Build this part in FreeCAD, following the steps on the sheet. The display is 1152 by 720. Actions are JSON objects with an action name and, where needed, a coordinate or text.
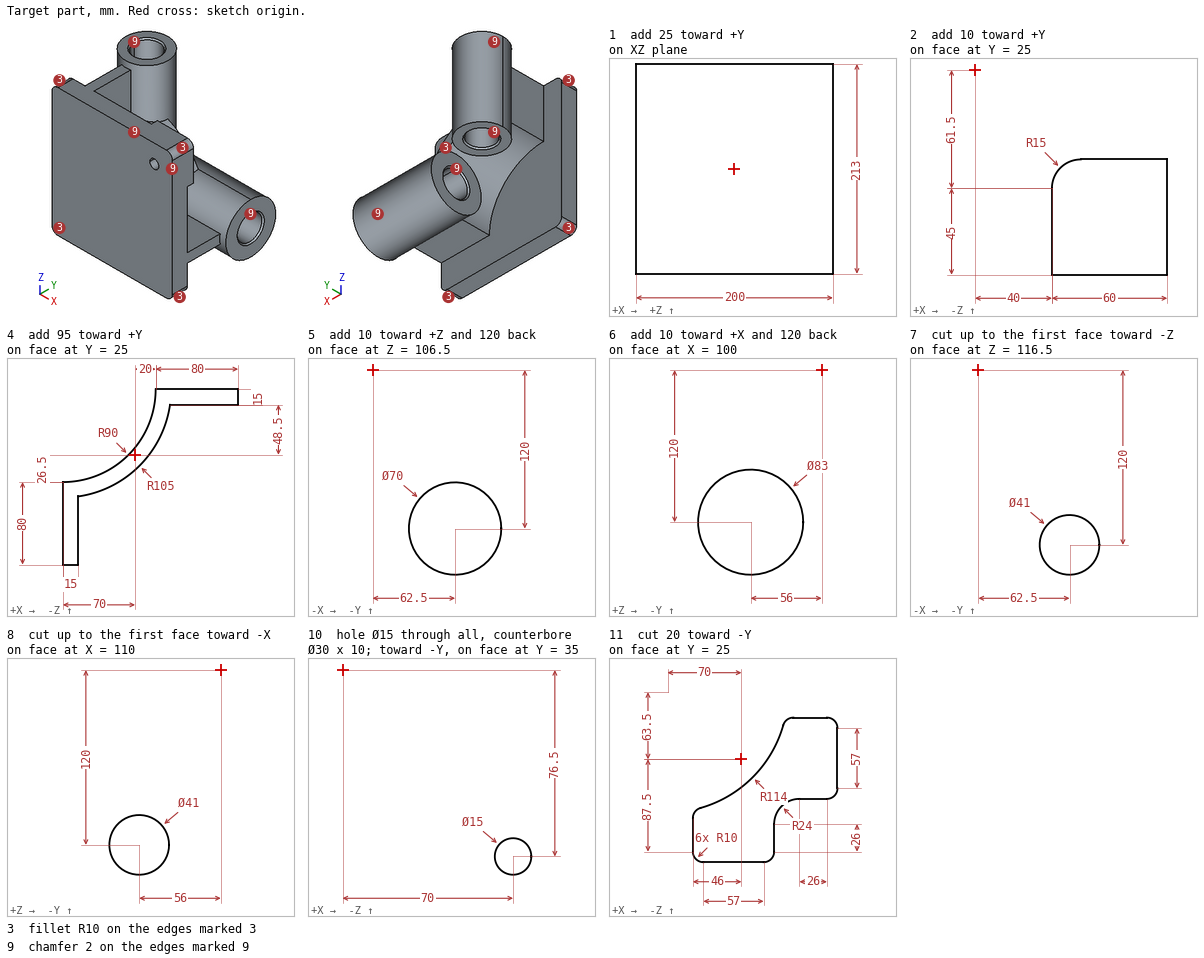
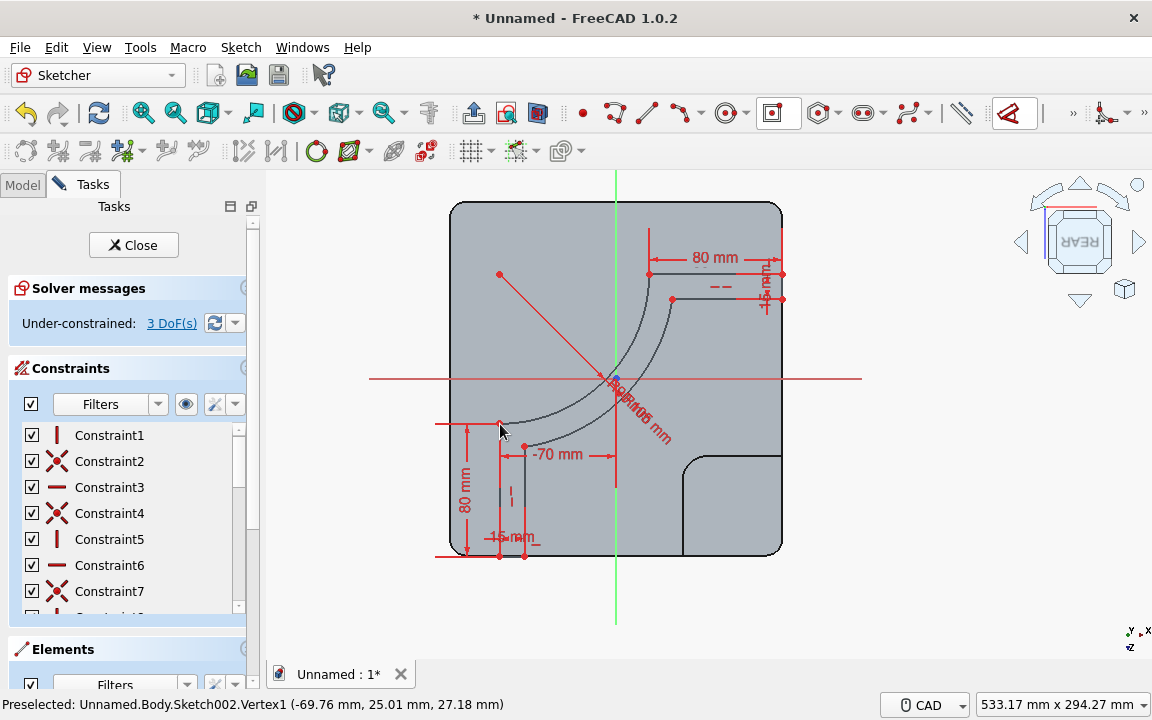
{"action": "left_click", "coordinate": [649, 274]}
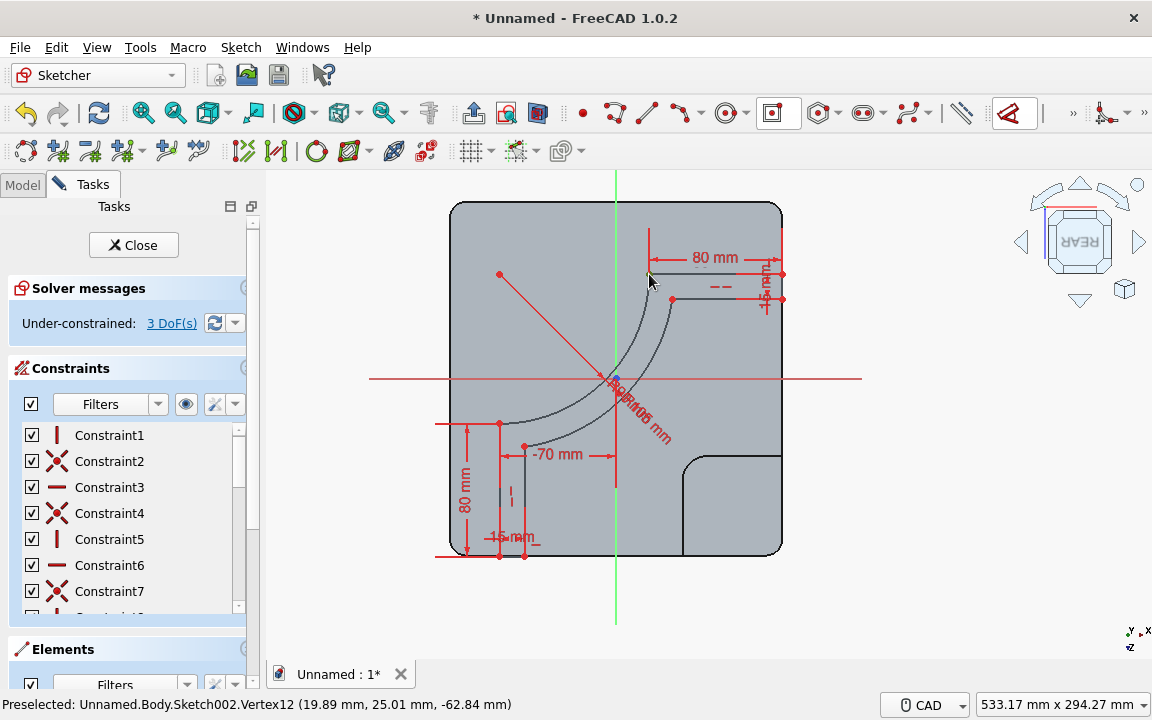
{"action": "left_click", "coordinate": [1032, 114]}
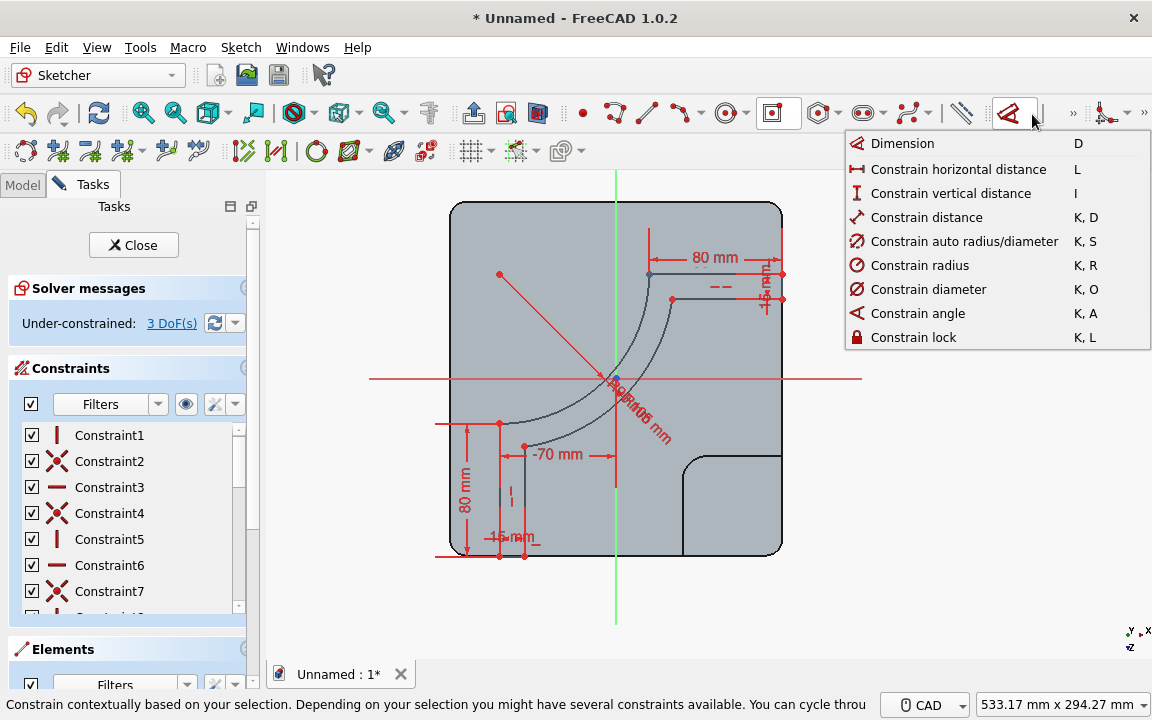
{"action": "left_click", "coordinate": [998, 169]}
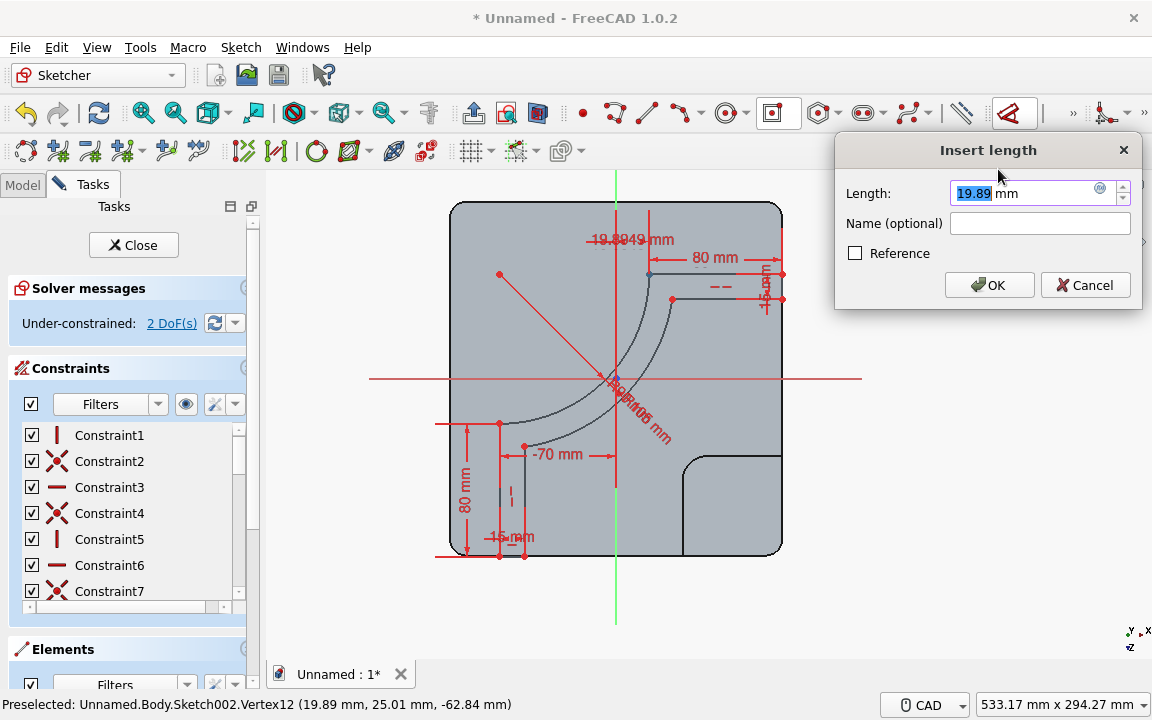
{"action": "type", "text": "20"}
{"action": "key", "text": "Return"}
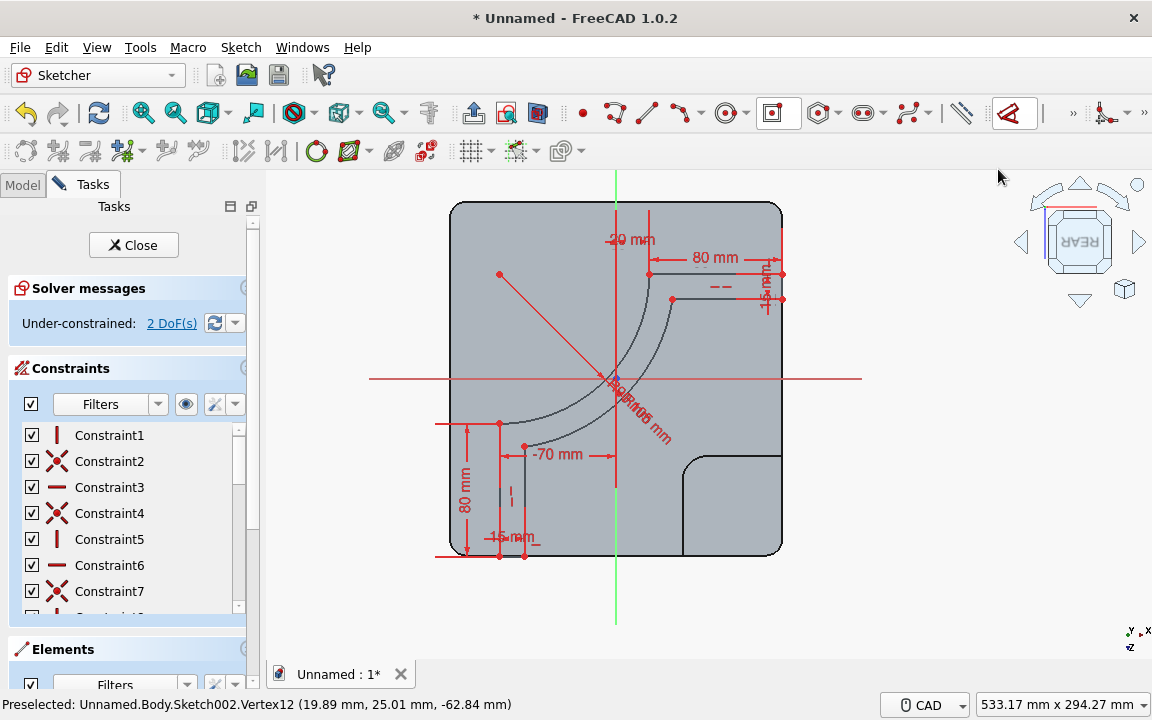
{"action": "left_click", "coordinate": [500, 424]}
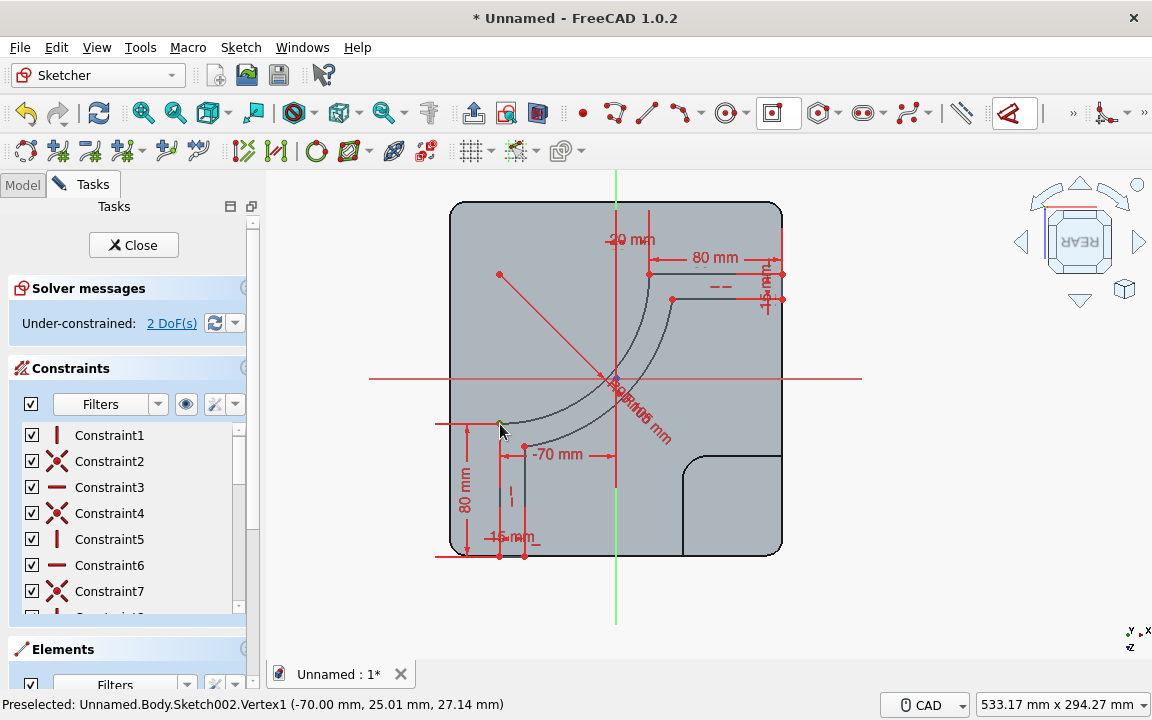
{"action": "left_click", "coordinate": [1032, 114]}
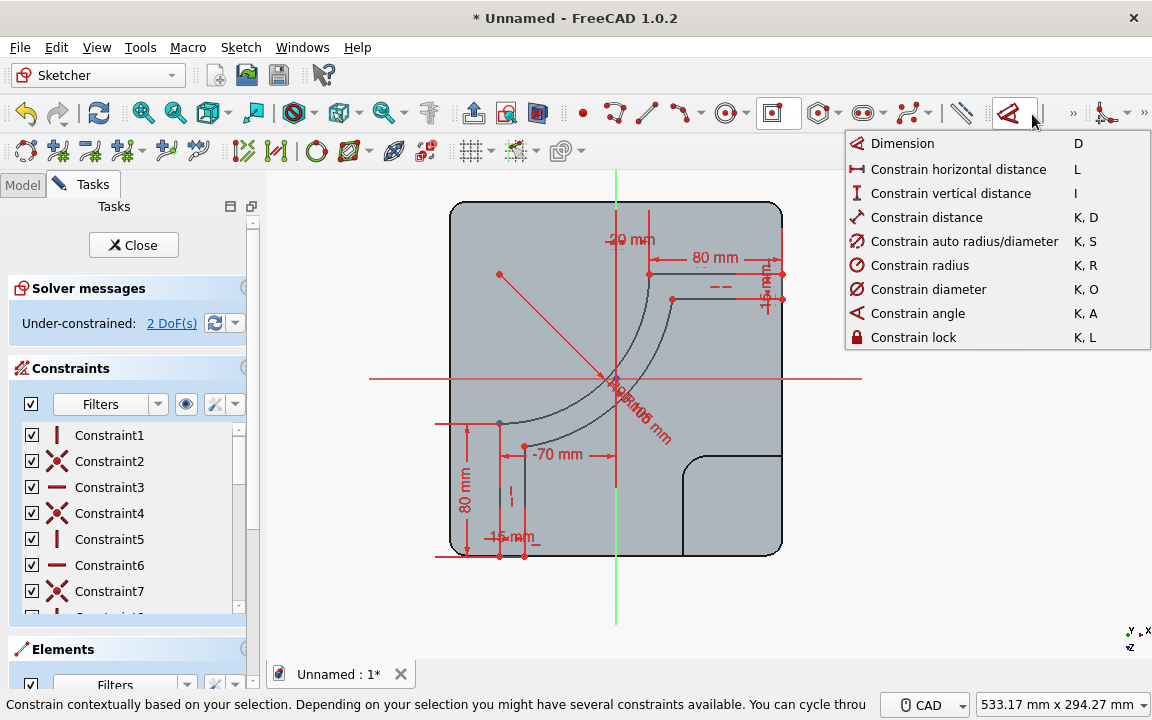
{"action": "left_click", "coordinate": [998, 193]}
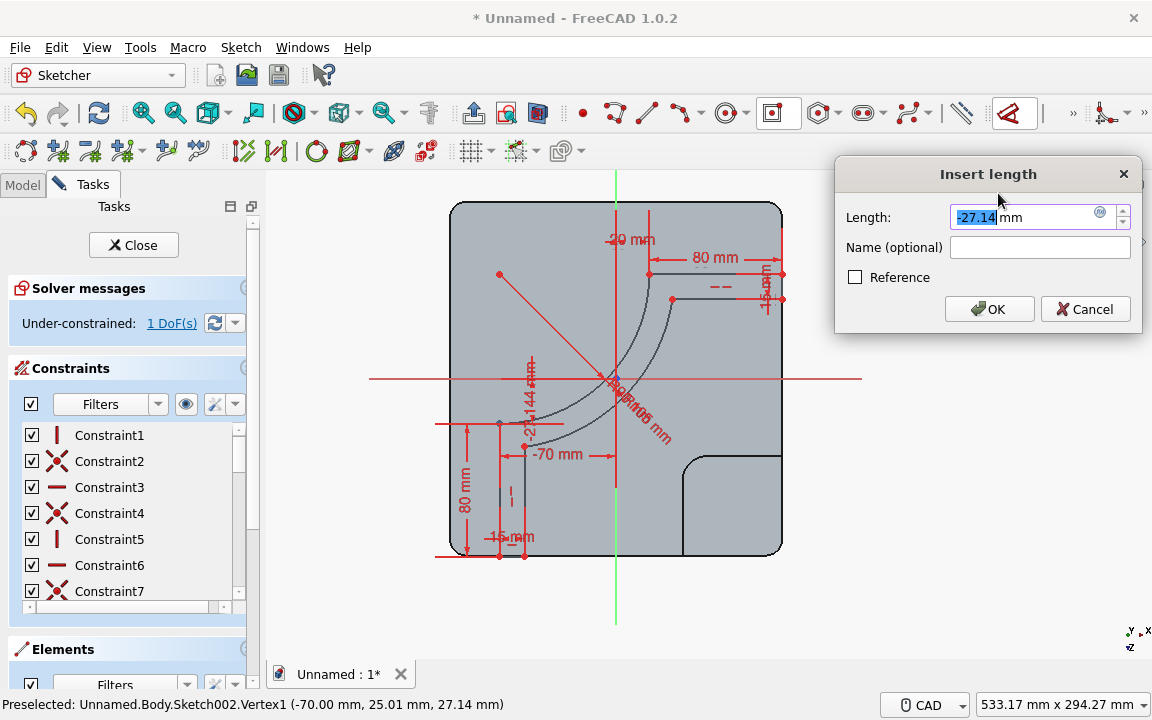
{"action": "type", "text": "-26.5"}
{"action": "key", "text": "Return"}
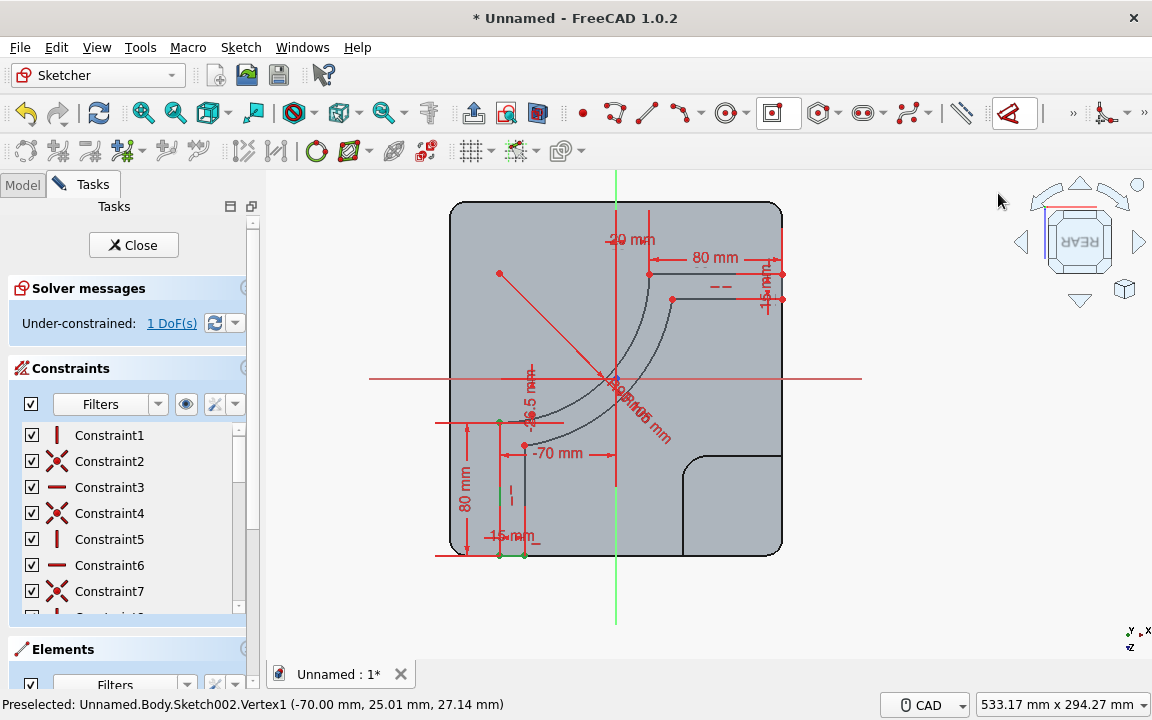
{"action": "left_click", "coordinate": [672, 299]}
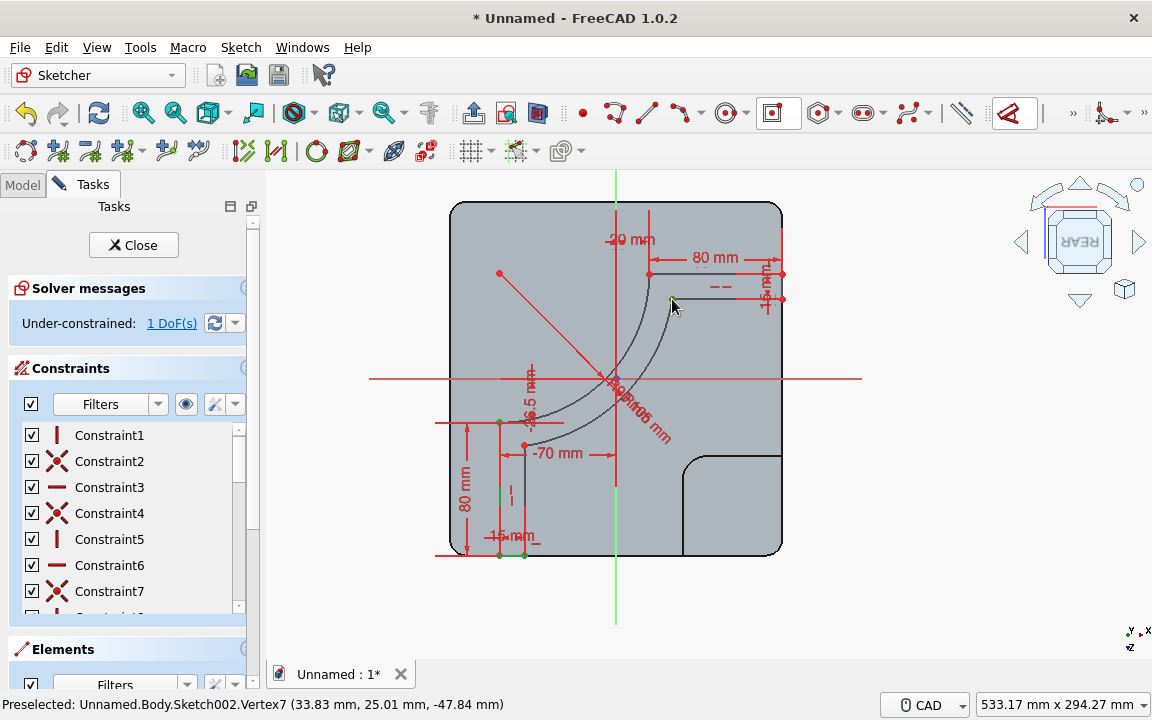
{"action": "key", "text": "i"}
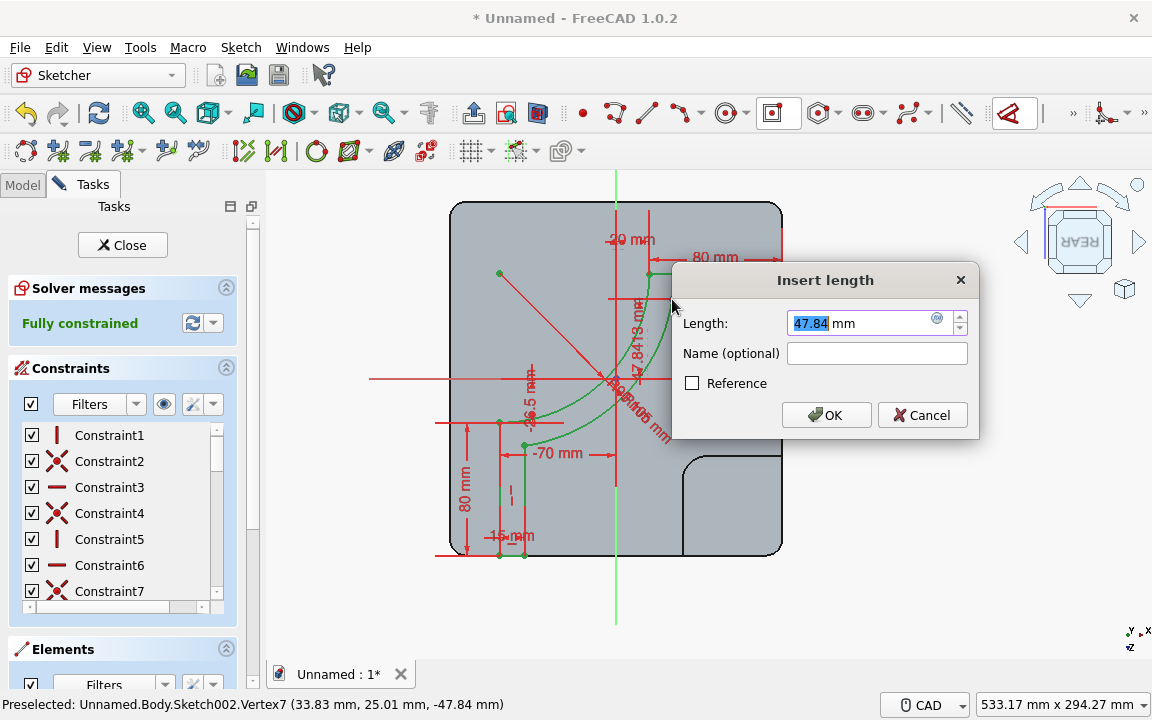
{"action": "type", "text": "48.5"}
{"action": "key", "text": "Return"}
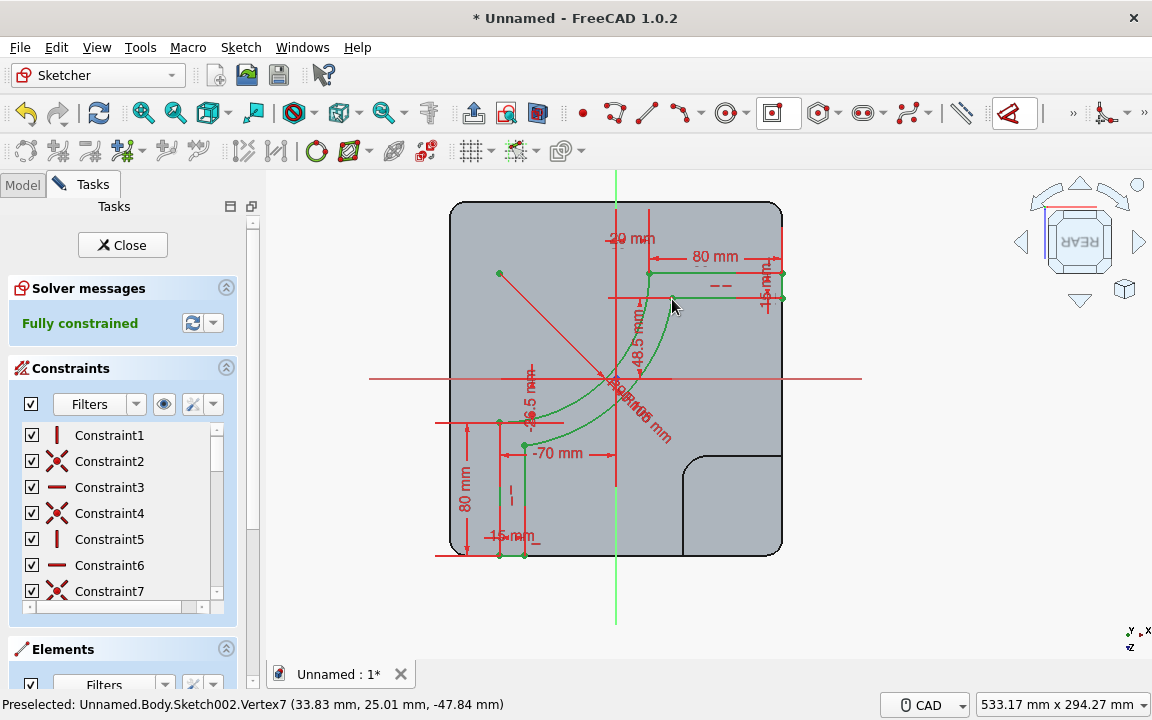
{"action": "left_click", "coordinate": [123, 245]}